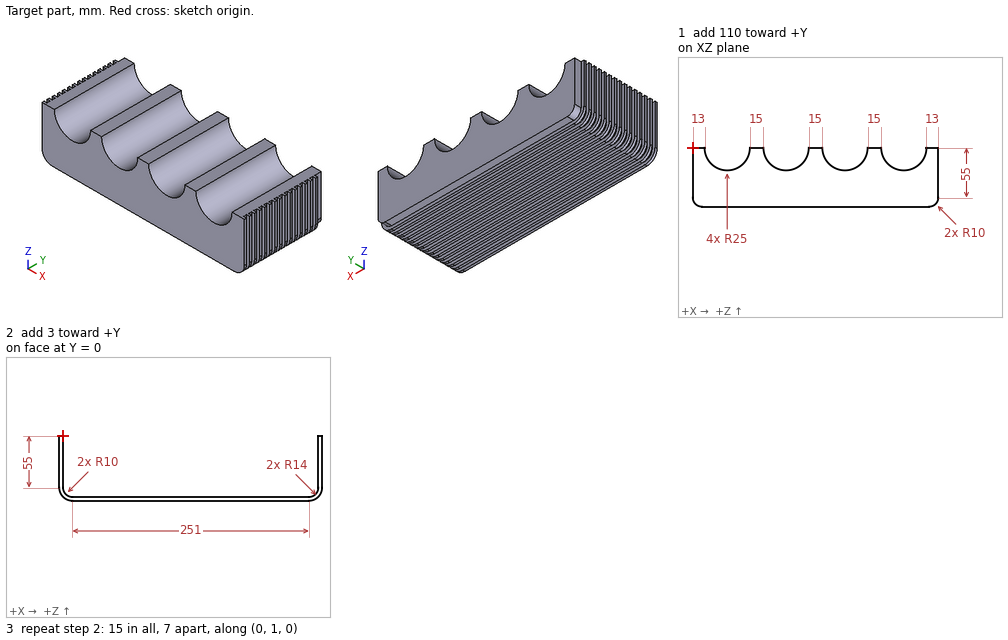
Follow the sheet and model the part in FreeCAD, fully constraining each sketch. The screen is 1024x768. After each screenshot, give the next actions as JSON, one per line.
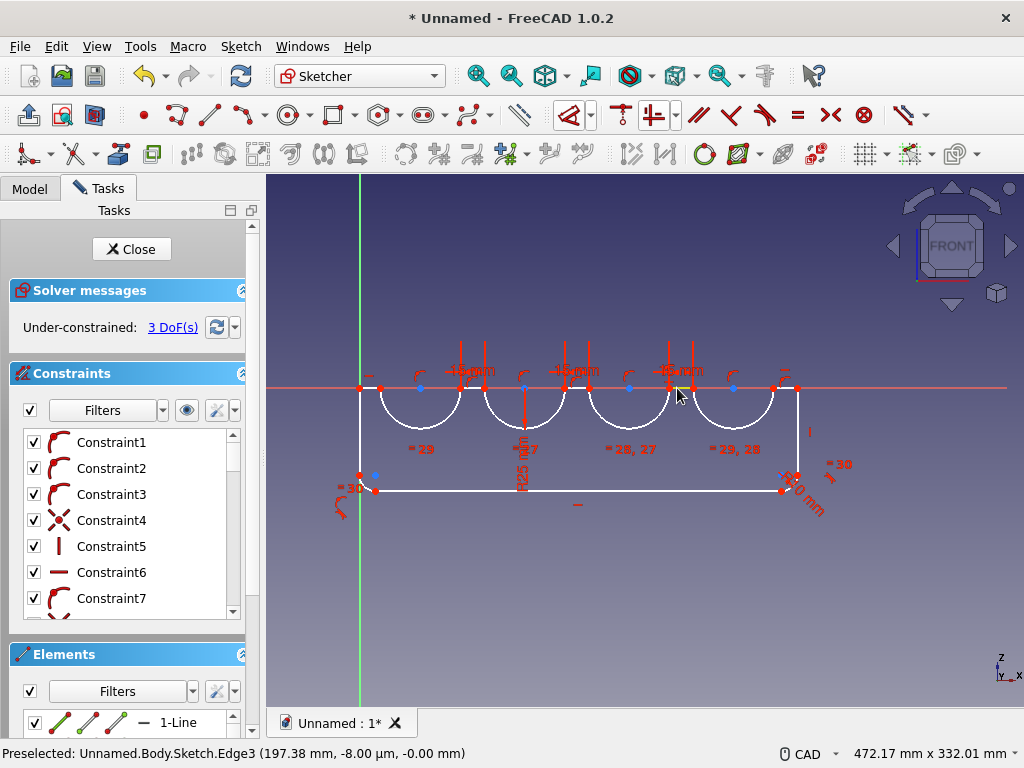
{"action": "scroll", "coordinate": [781, 388], "scroll_direction": "up", "scroll_amount": 4}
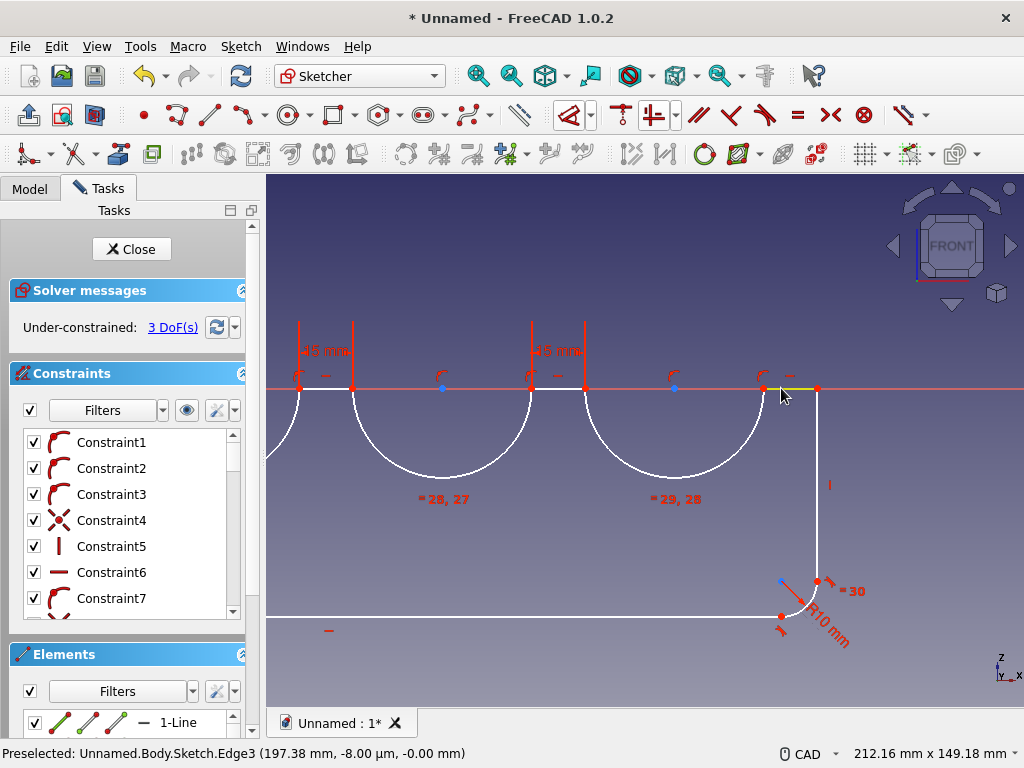
{"action": "left_click", "coordinate": [780, 389]}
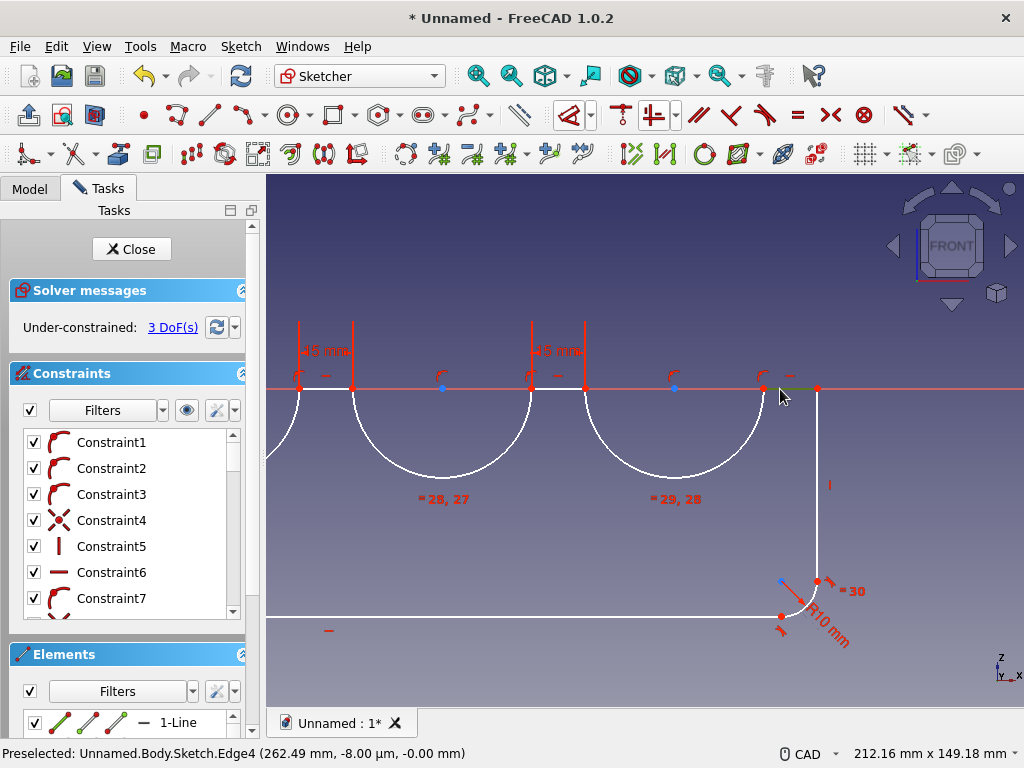
{"action": "key", "text": "l"}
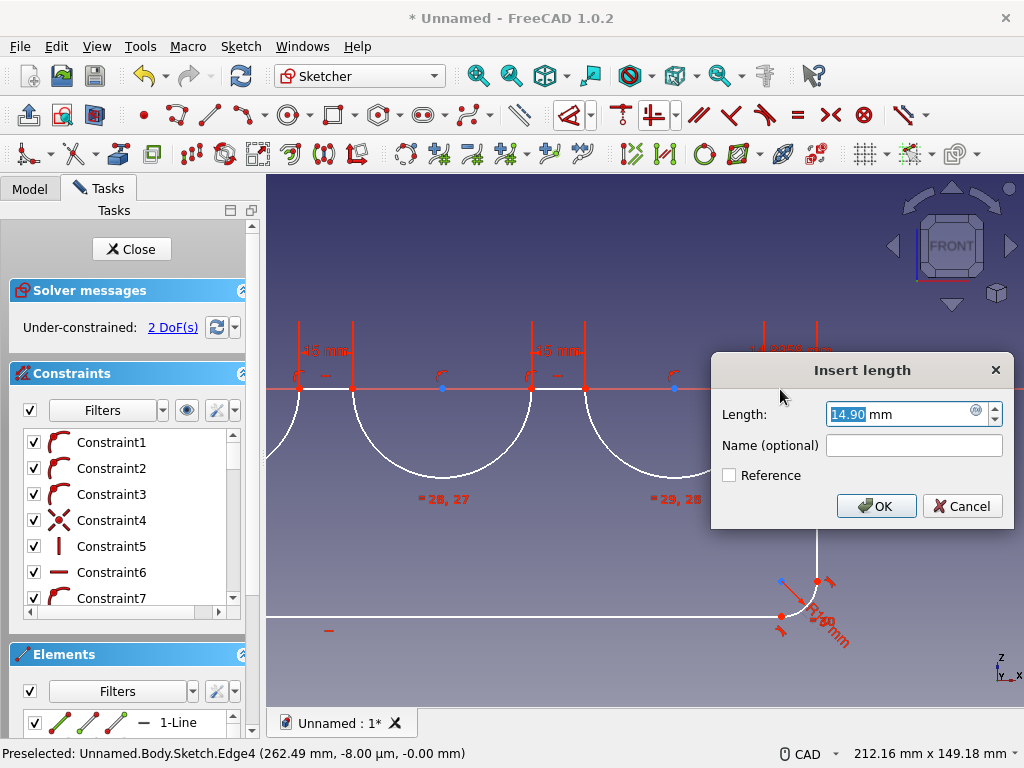
{"action": "type", "text": "13"}
{"action": "key", "text": "Return"}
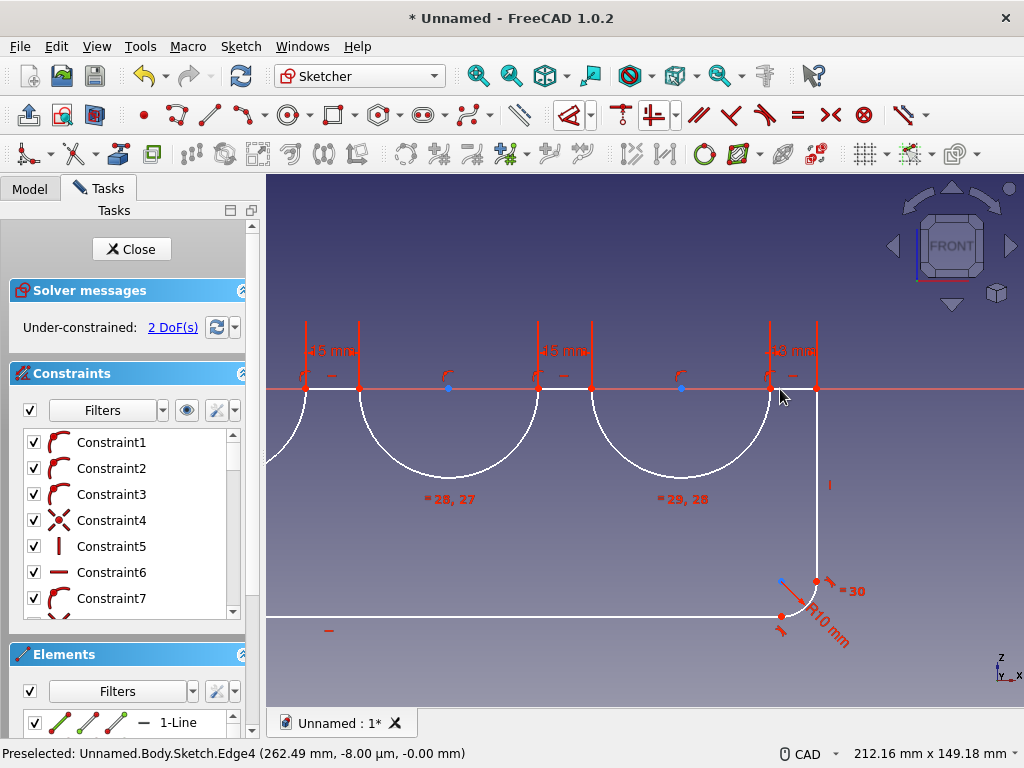
{"action": "left_click", "coordinate": [817, 446]}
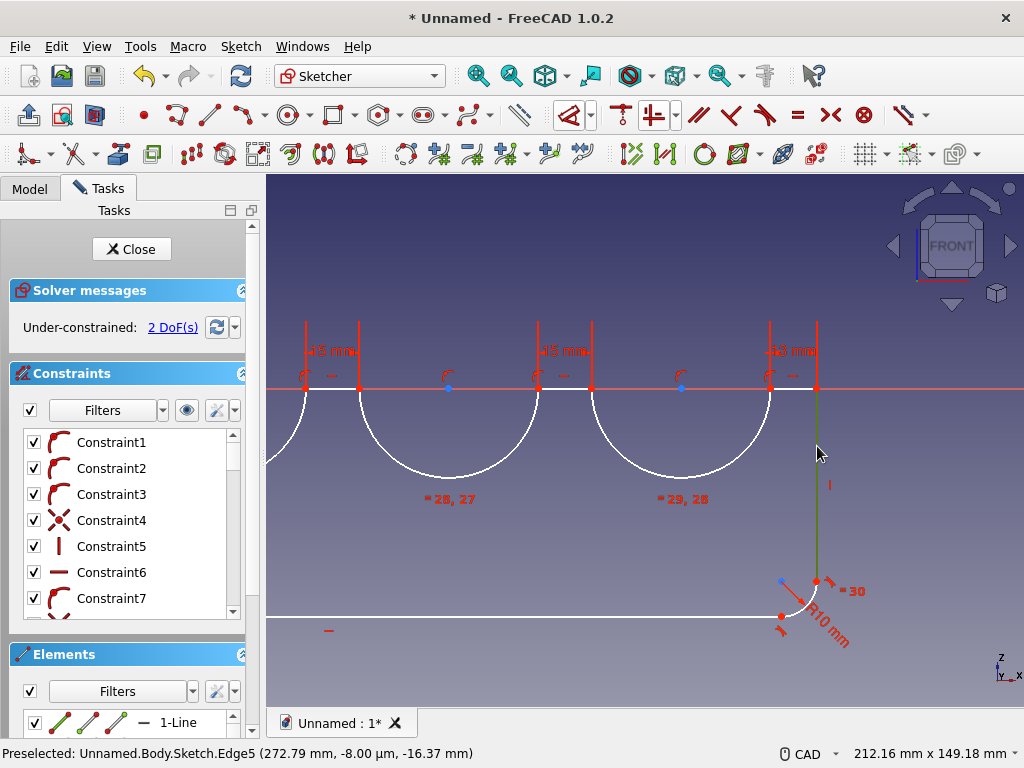
{"action": "key", "text": "i"}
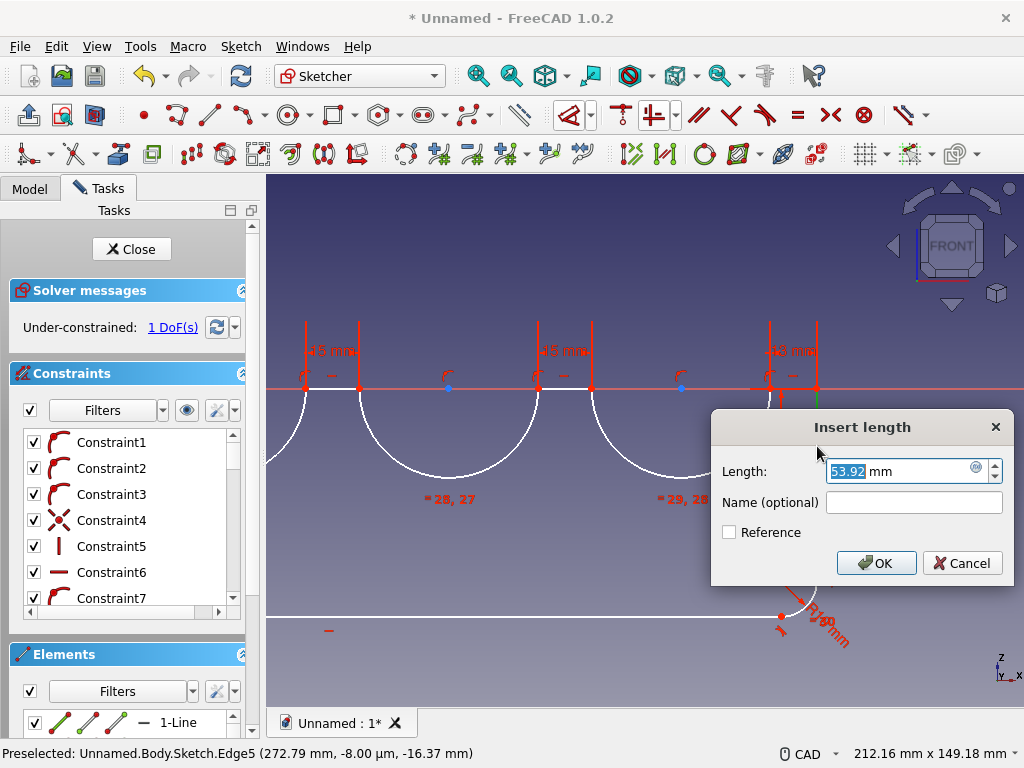
{"action": "type", "text": "55"}
{"action": "key", "text": "Return"}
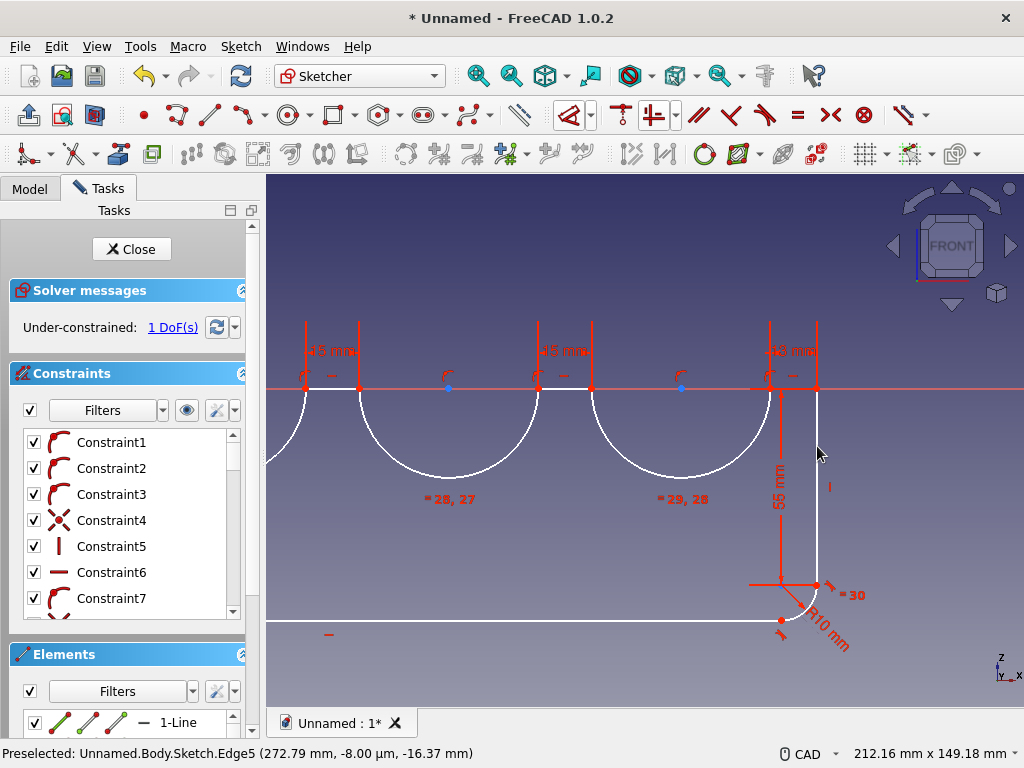
{"action": "scroll", "coordinate": [781, 388], "scroll_direction": "down", "scroll_amount": 4}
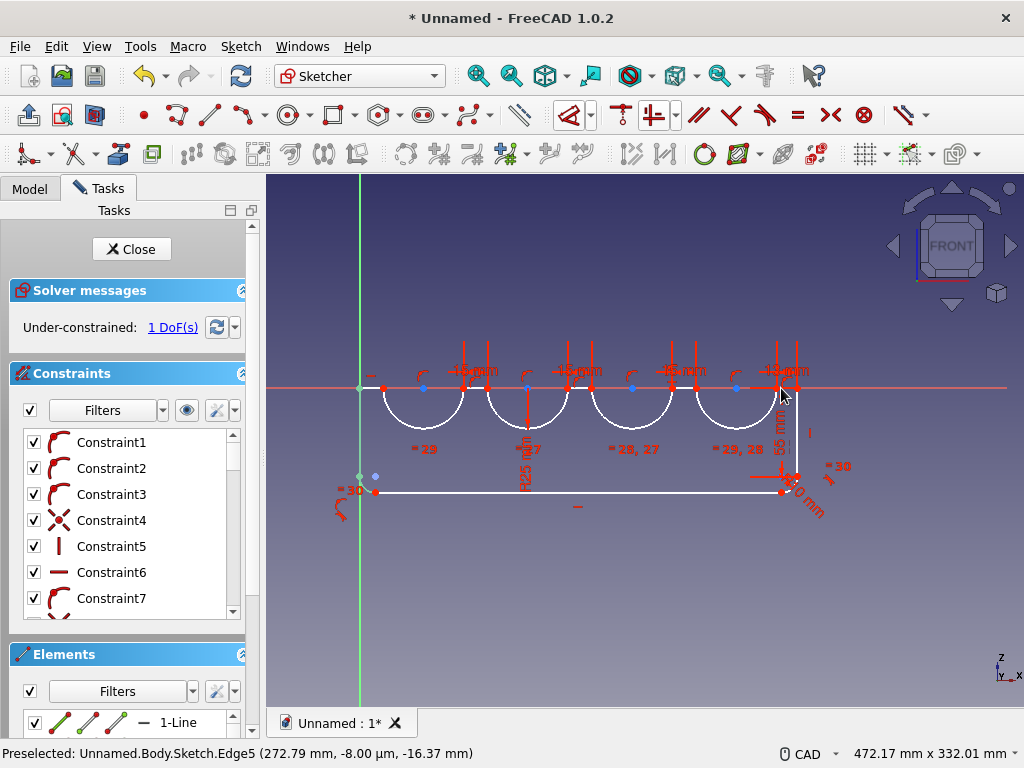
{"action": "scroll", "coordinate": [367, 388], "scroll_direction": "up", "scroll_amount": 4}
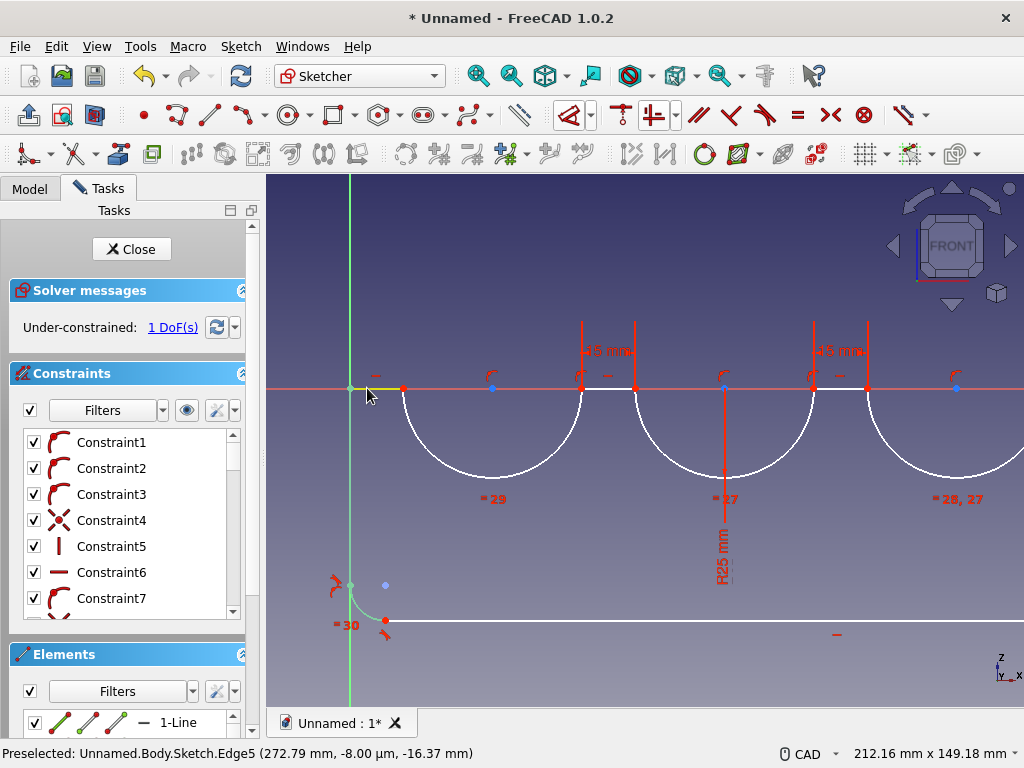
{"action": "left_click", "coordinate": [366, 389]}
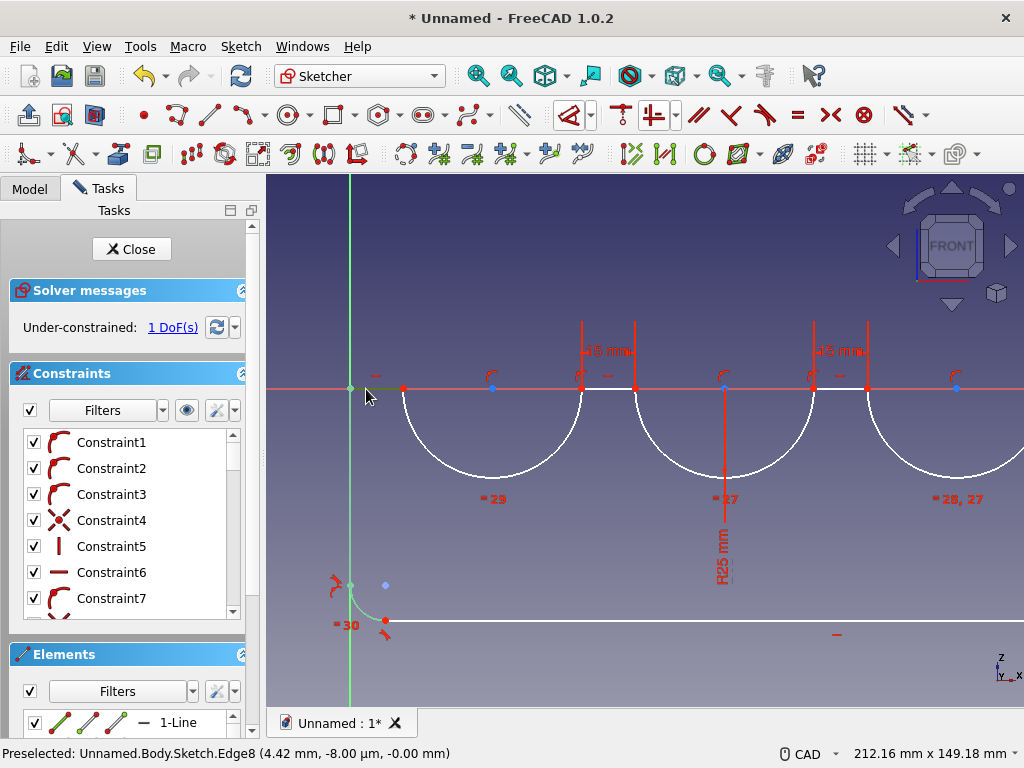
{"action": "key", "text": "l"}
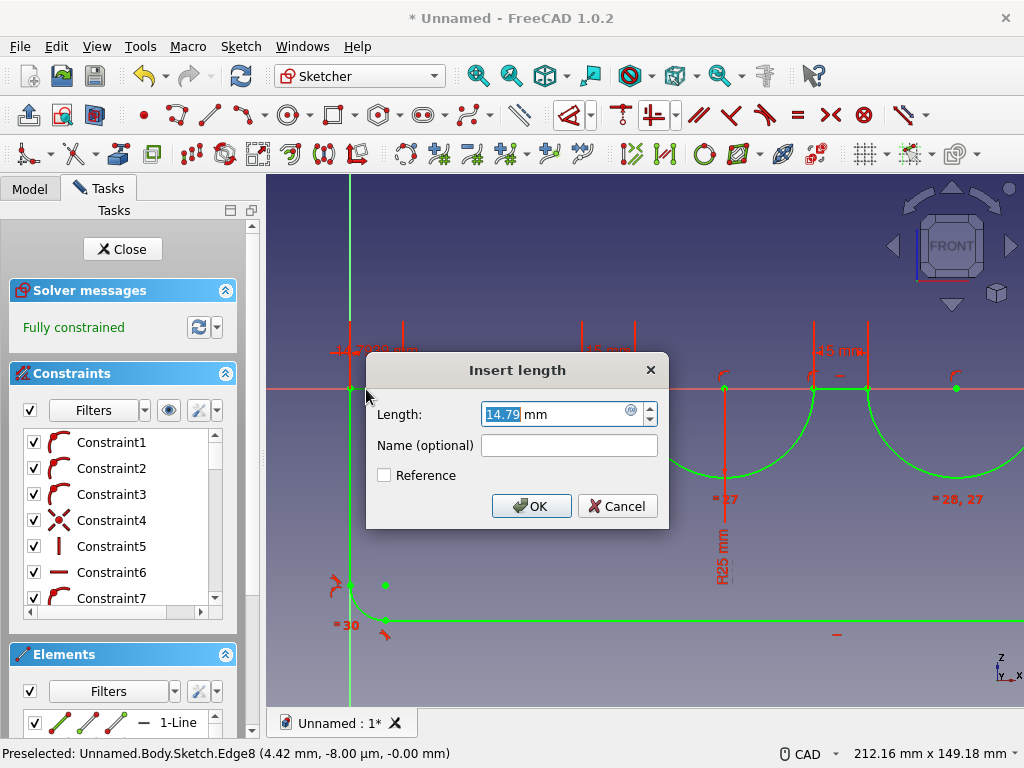
{"action": "type", "text": "13"}
{"action": "key", "text": "Return"}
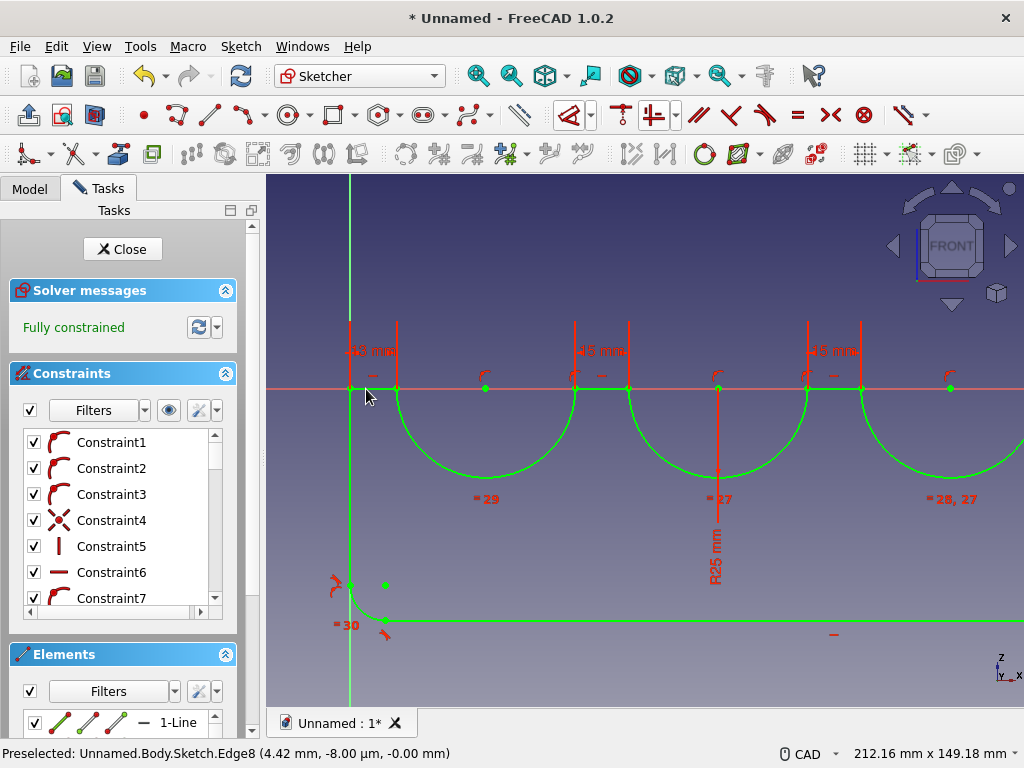
{"action": "left_click", "coordinate": [123, 249]}